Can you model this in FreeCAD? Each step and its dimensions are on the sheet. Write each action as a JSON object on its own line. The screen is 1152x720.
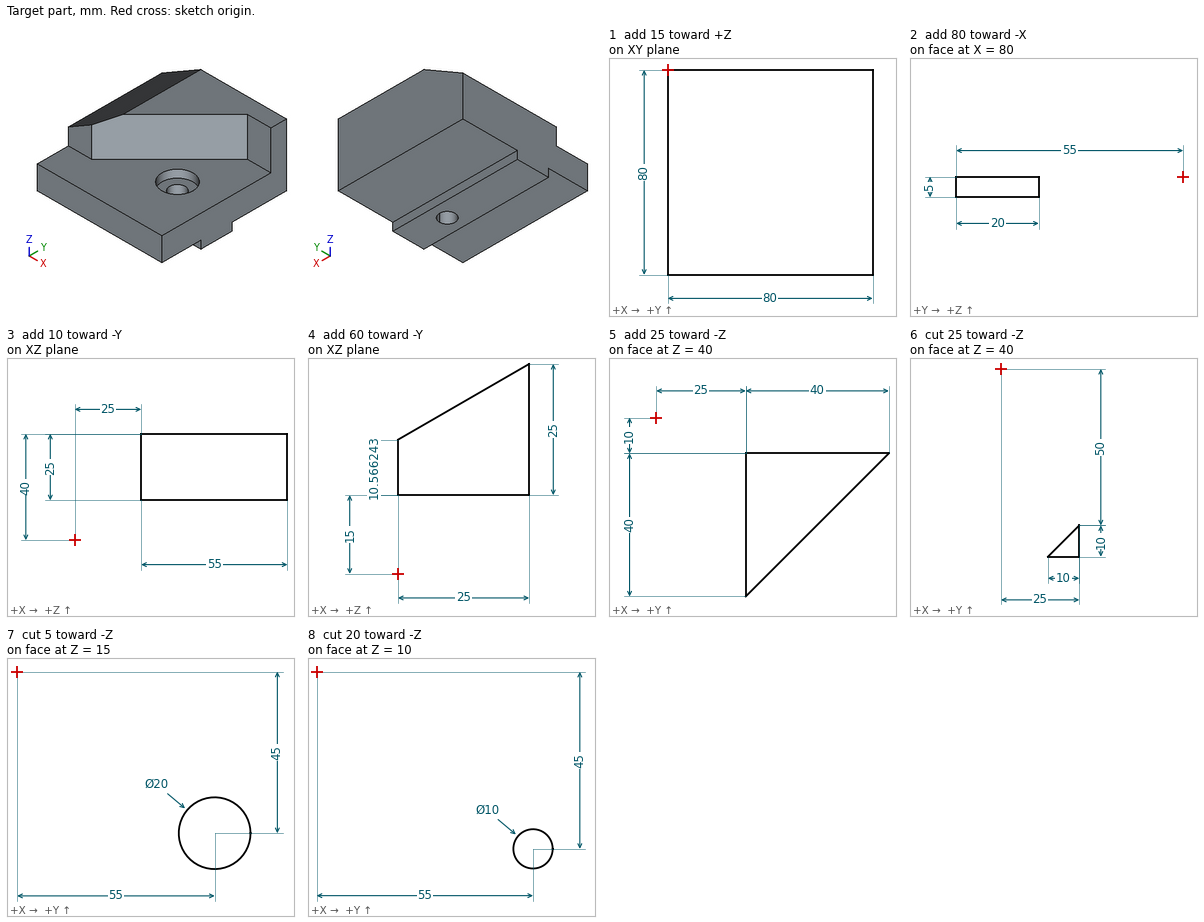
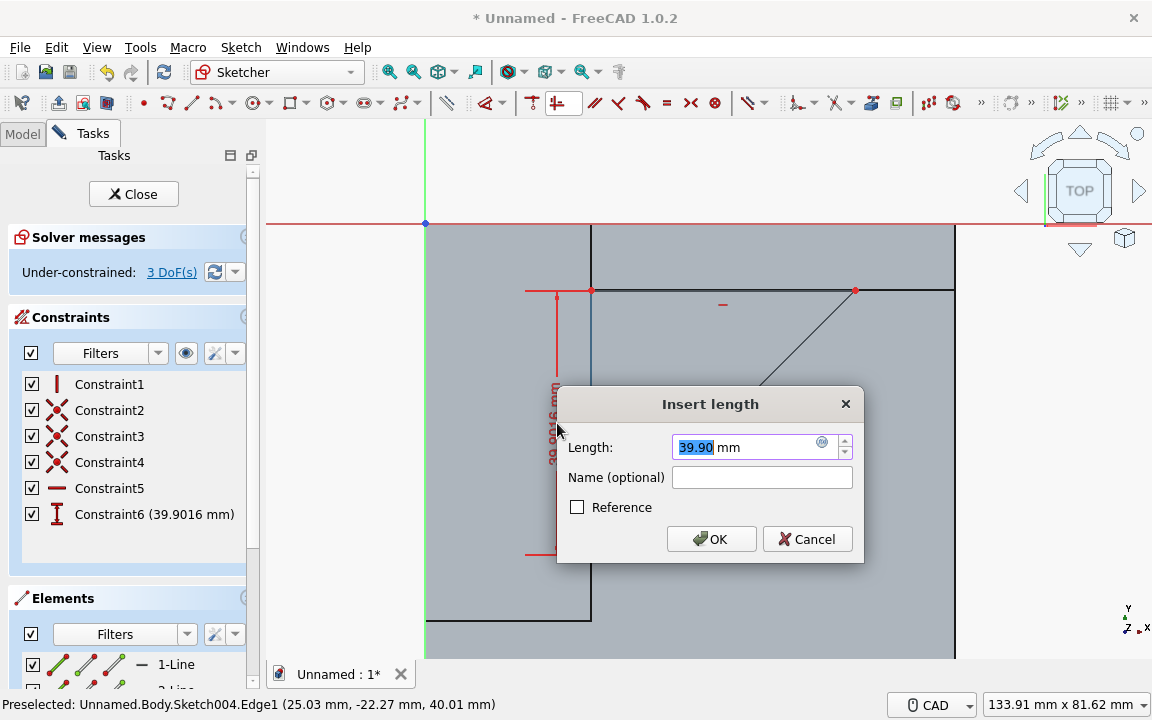
{"action": "type", "text": "40"}
{"action": "key", "text": "Return"}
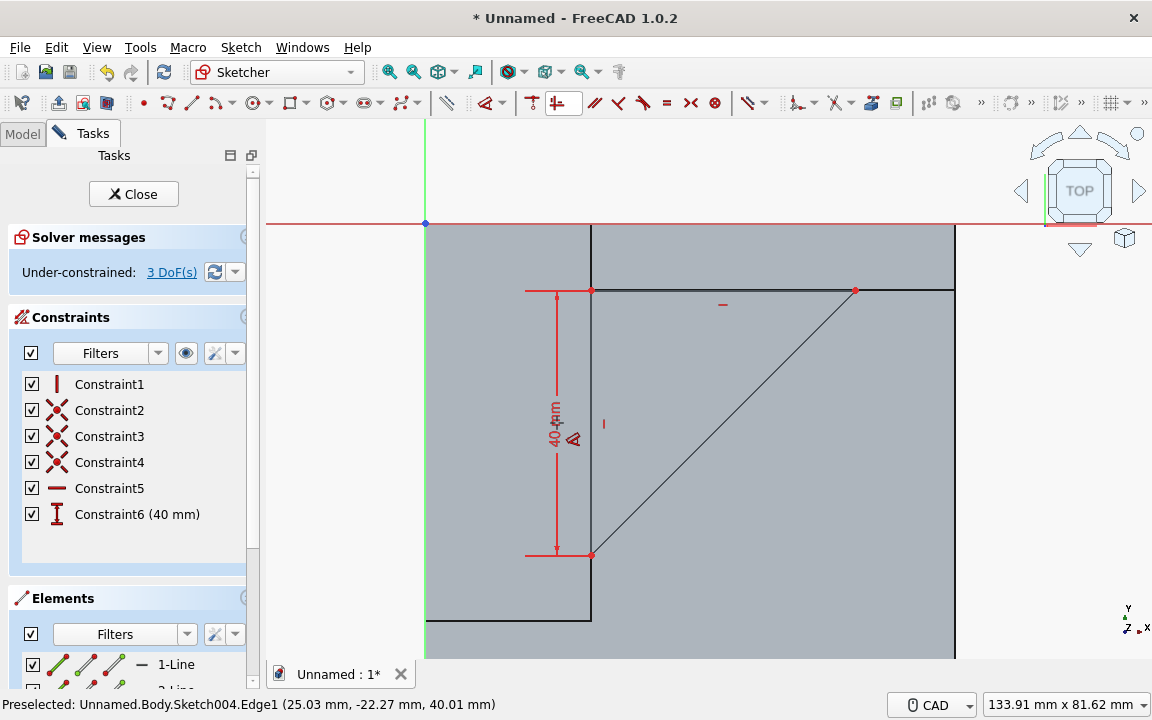
{"action": "left_click", "coordinate": [776, 291]}
{"action": "left_click", "coordinate": [723, 257]}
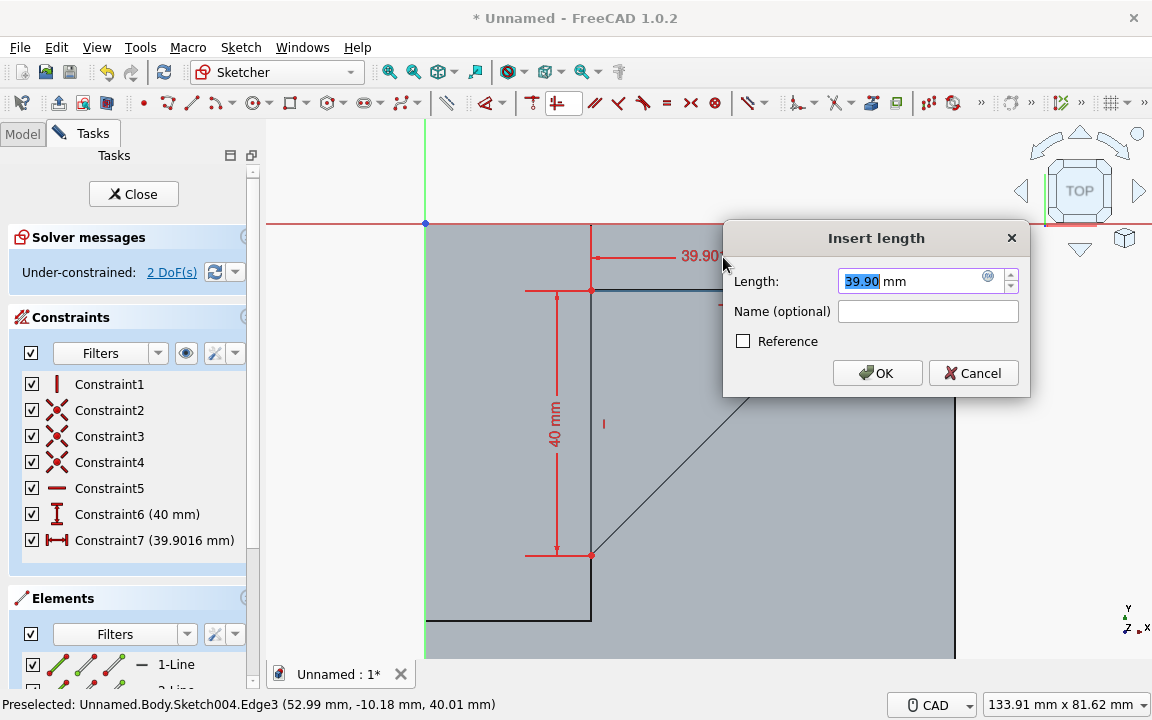
{"action": "type", "text": "40"}
{"action": "key", "text": "Return"}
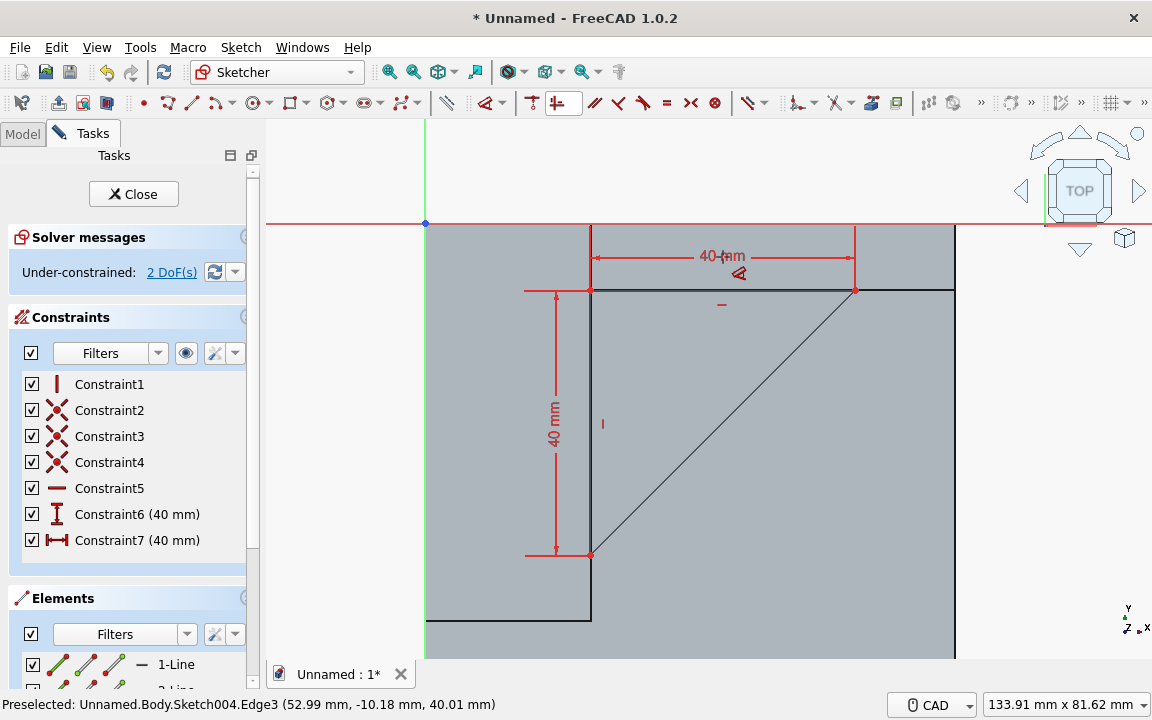
{"action": "left_click", "coordinate": [590, 291]}
{"action": "left_click", "coordinate": [508, 190]}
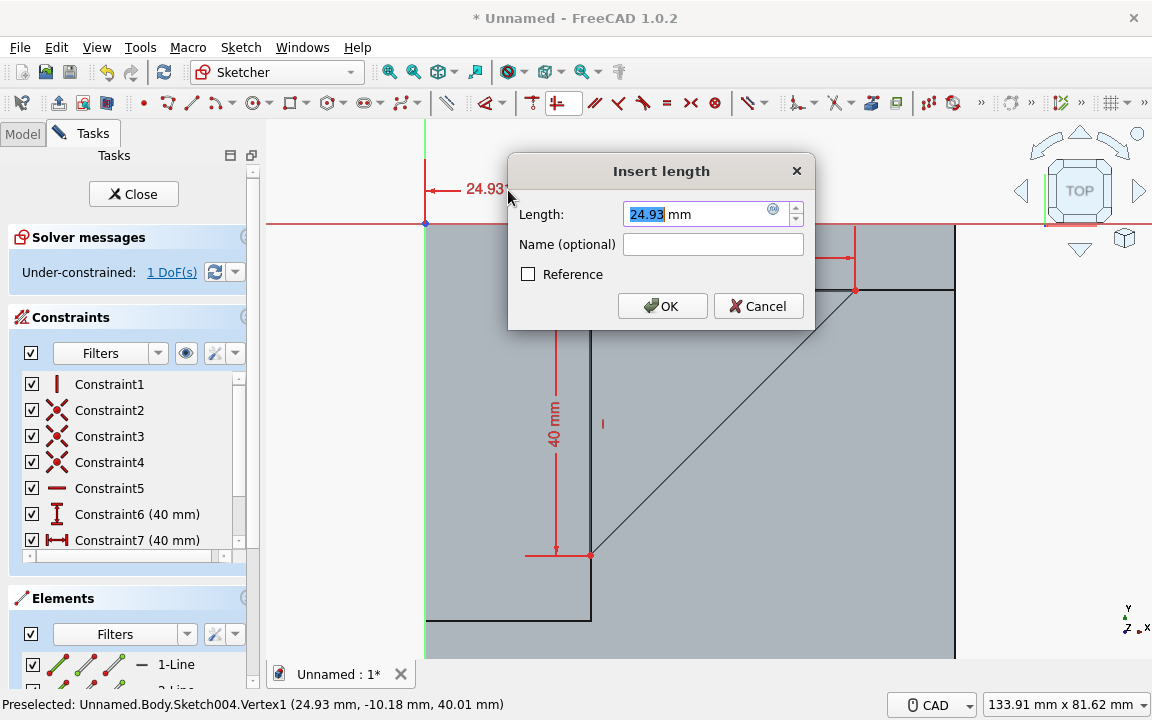
{"action": "type", "text": "25"}
{"action": "key", "text": "Return"}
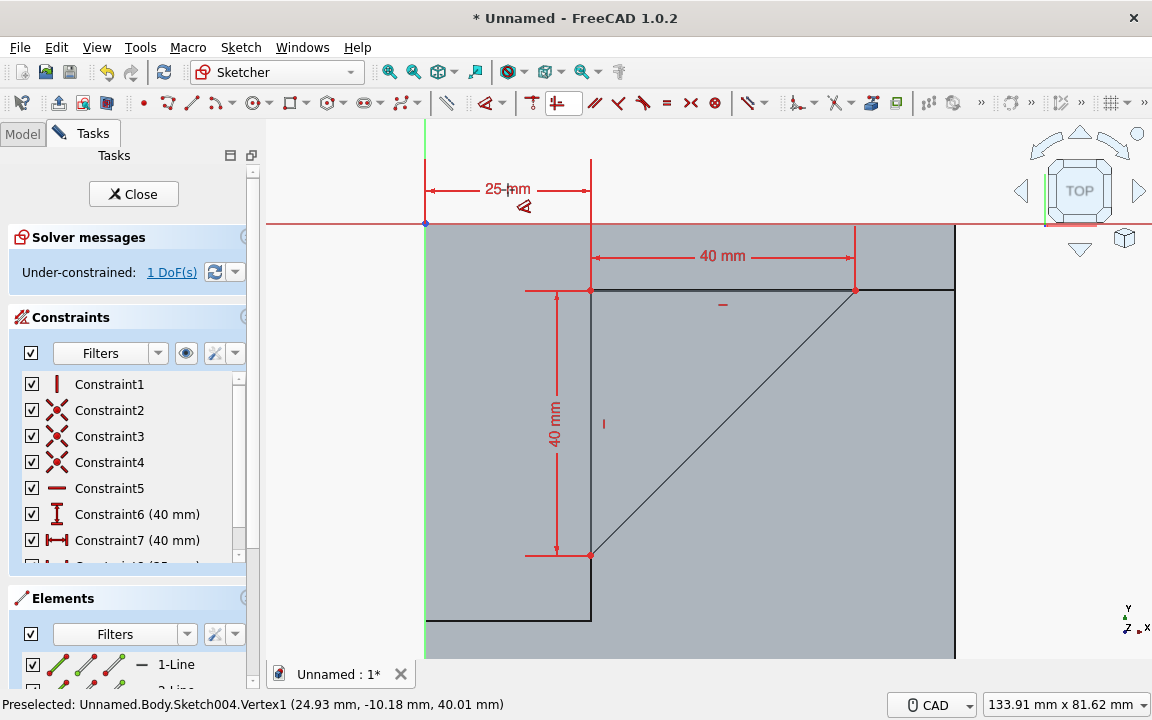
{"action": "left_click", "coordinate": [591, 291]}
{"action": "left_click", "coordinate": [391, 257]}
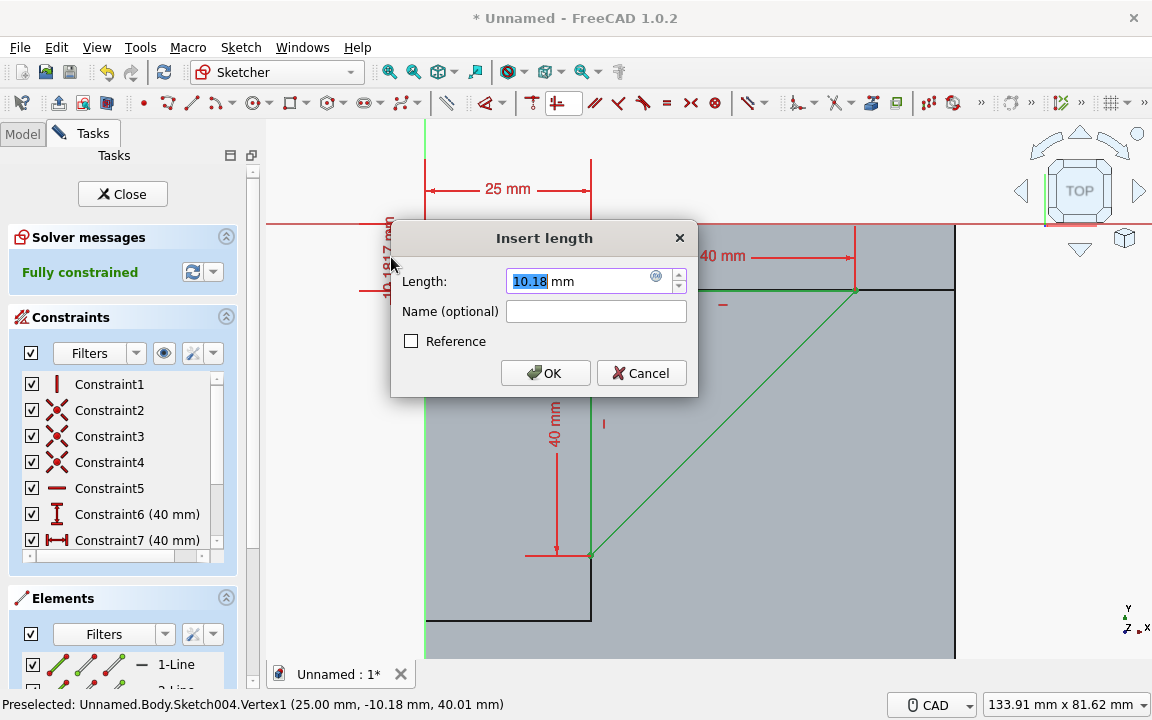
{"action": "type", "text": "10"}
{"action": "key", "text": "Return"}
{"action": "key", "text": "Escape"}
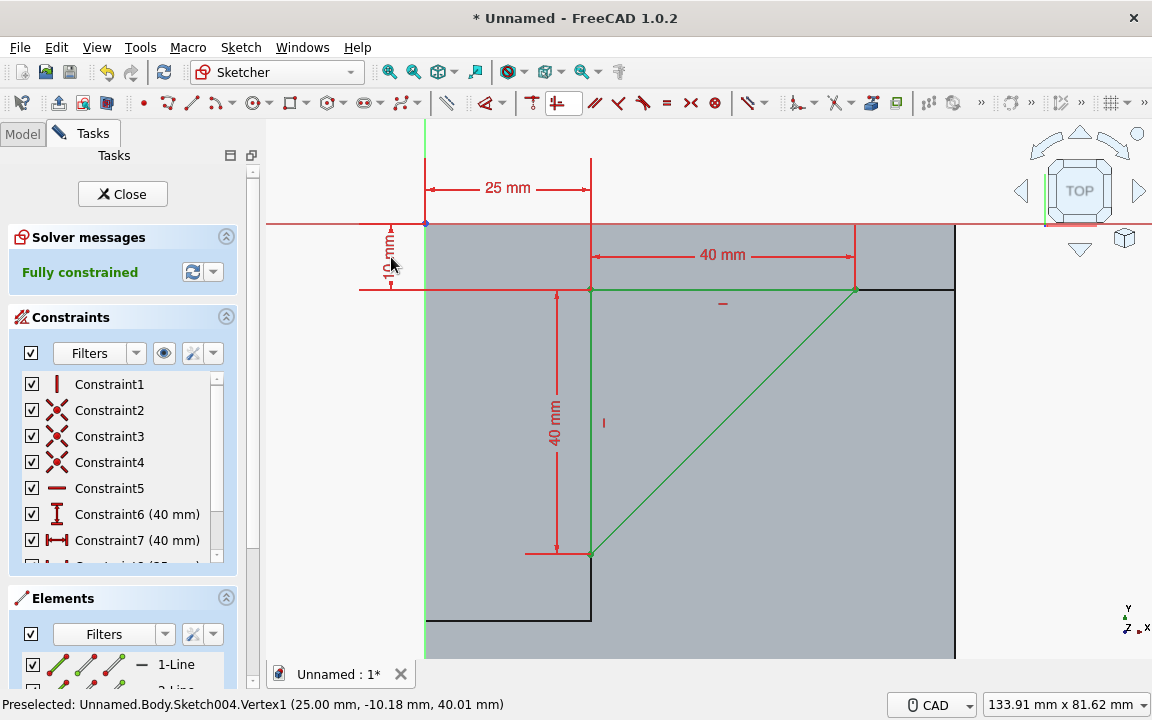
{"action": "left_click", "coordinate": [123, 194]}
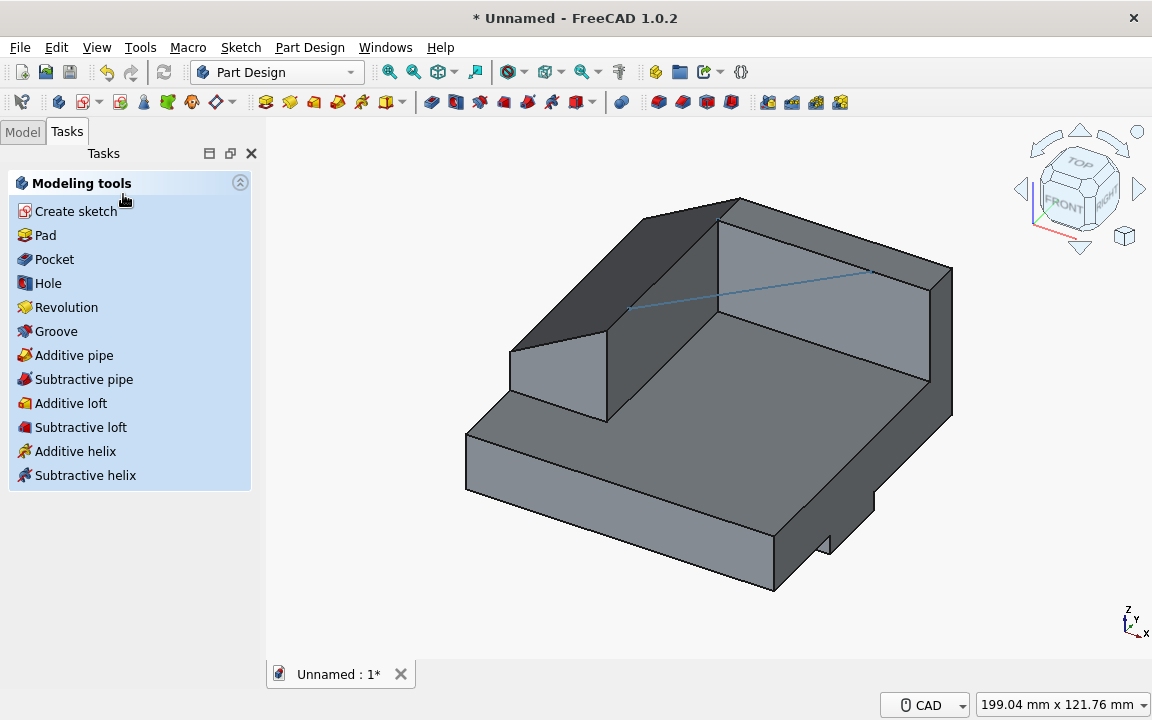
{"action": "left_click", "coordinate": [266, 102]}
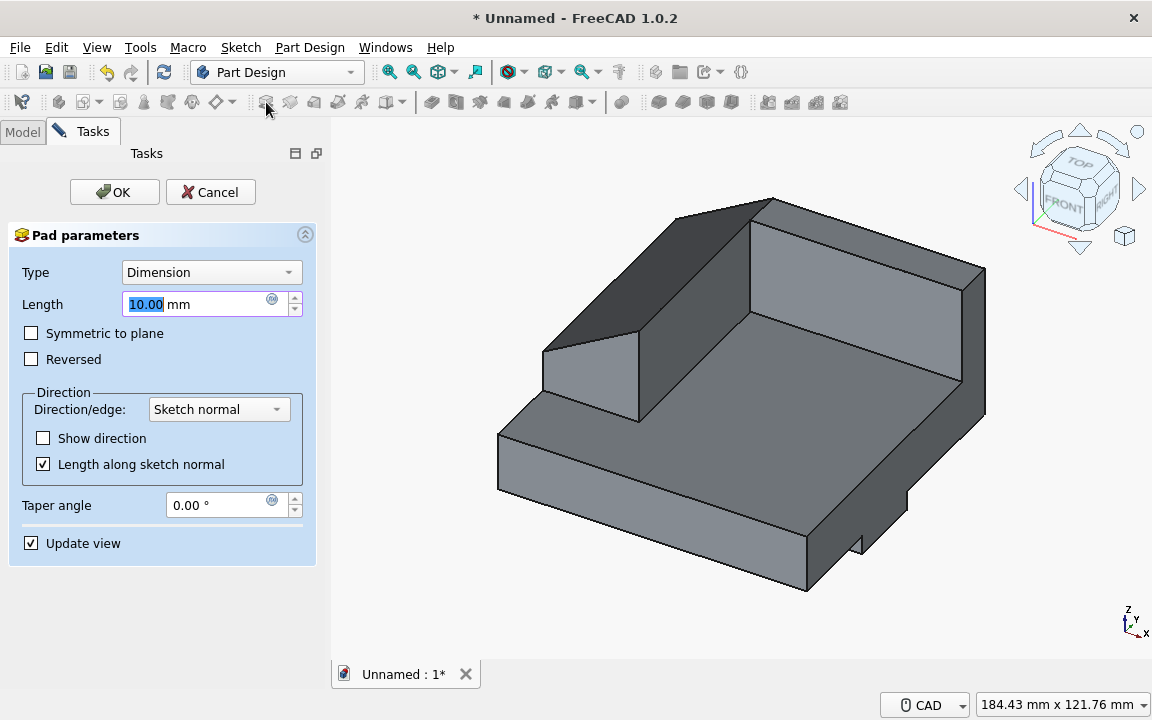
{"action": "type", "text": "25"}
{"action": "key", "text": "Tab"}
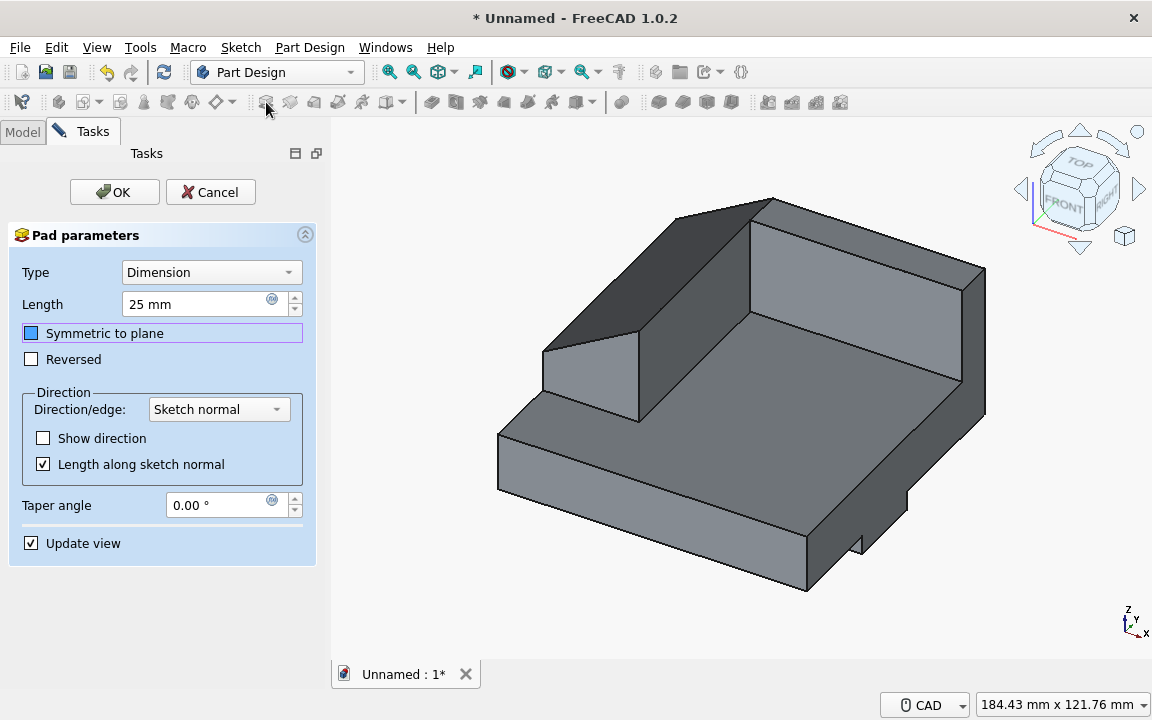
{"action": "left_click", "coordinate": [30, 359]}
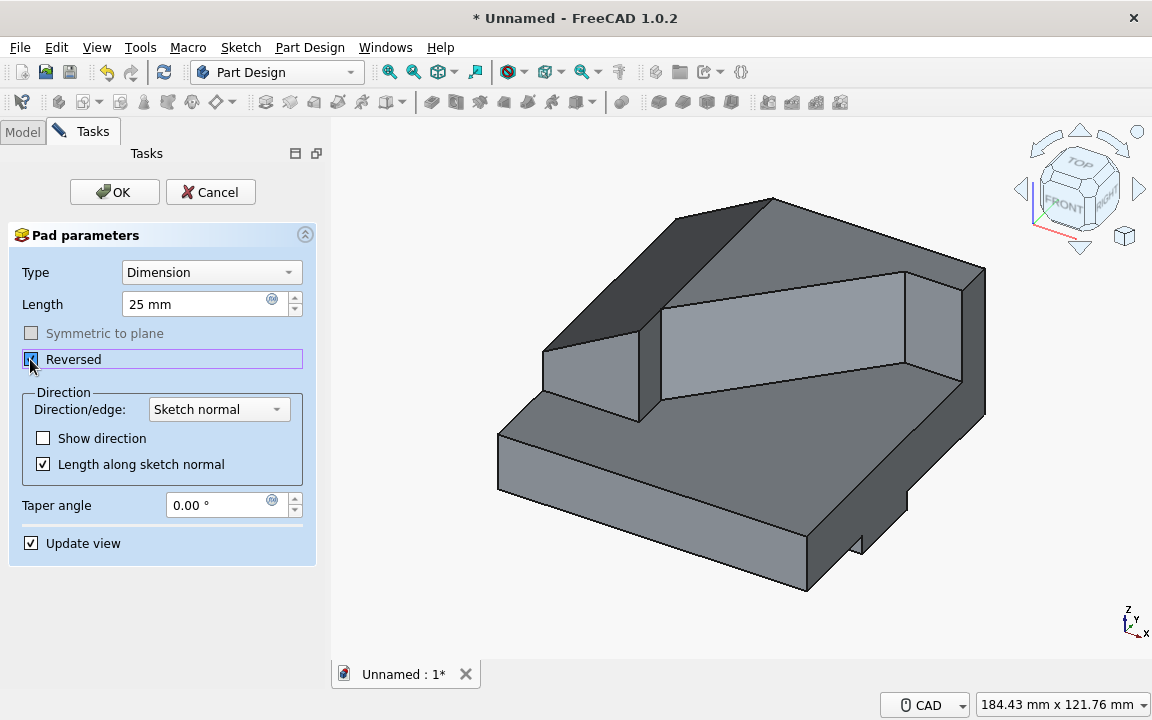
{"action": "left_click", "coordinate": [115, 192]}